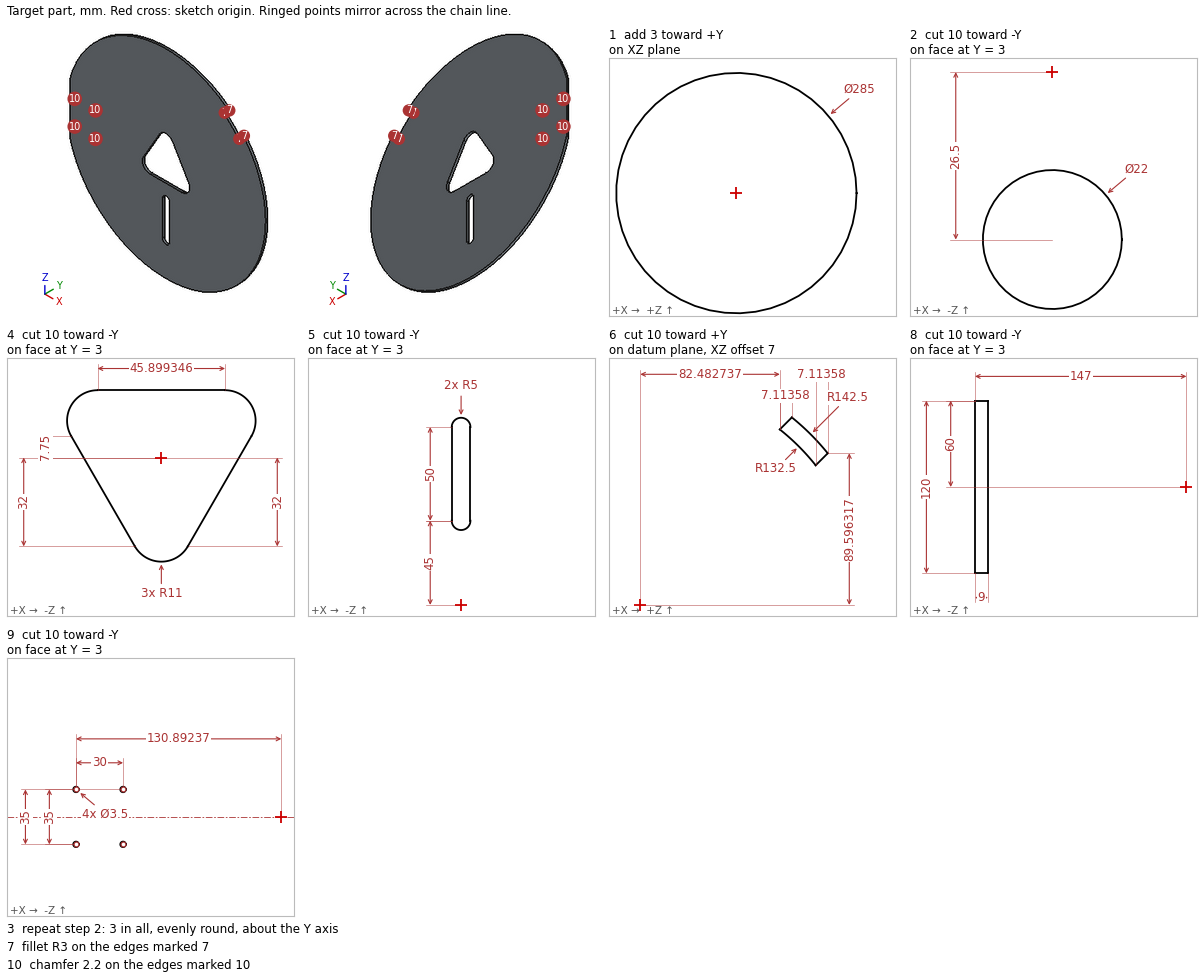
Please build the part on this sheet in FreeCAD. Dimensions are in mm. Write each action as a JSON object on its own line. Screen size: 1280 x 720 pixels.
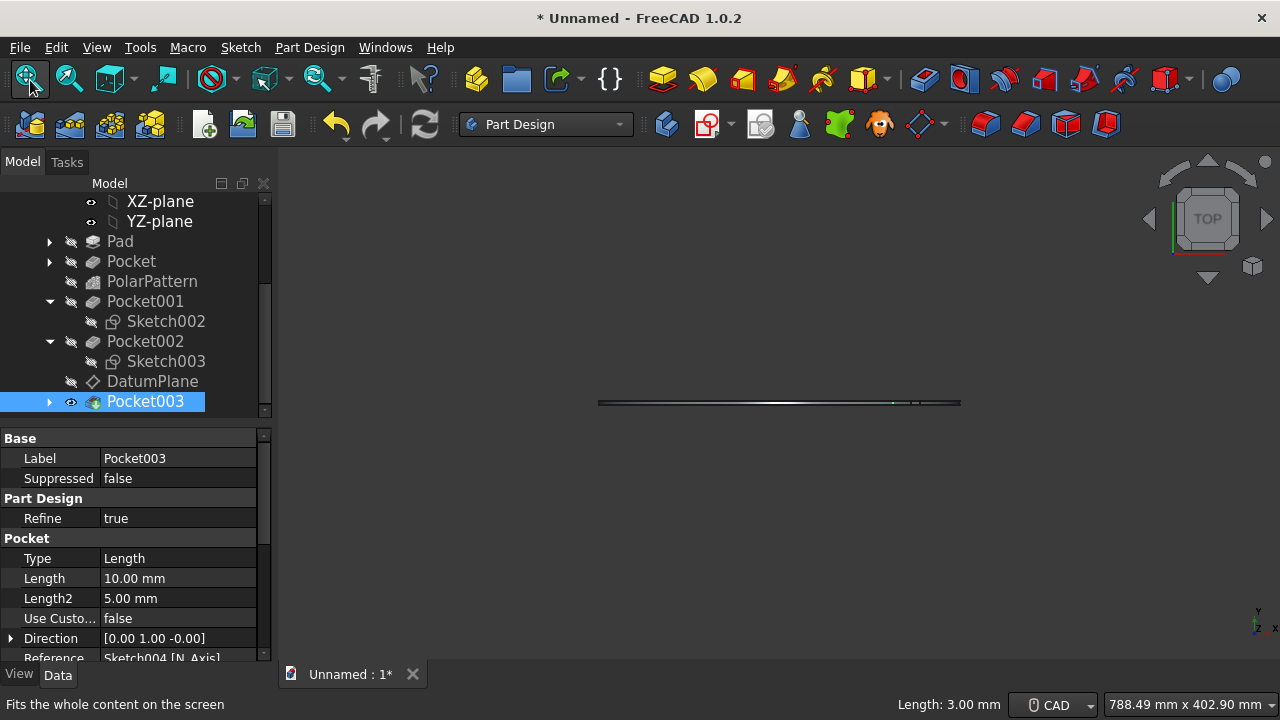
{"action": "key", "text": "1"}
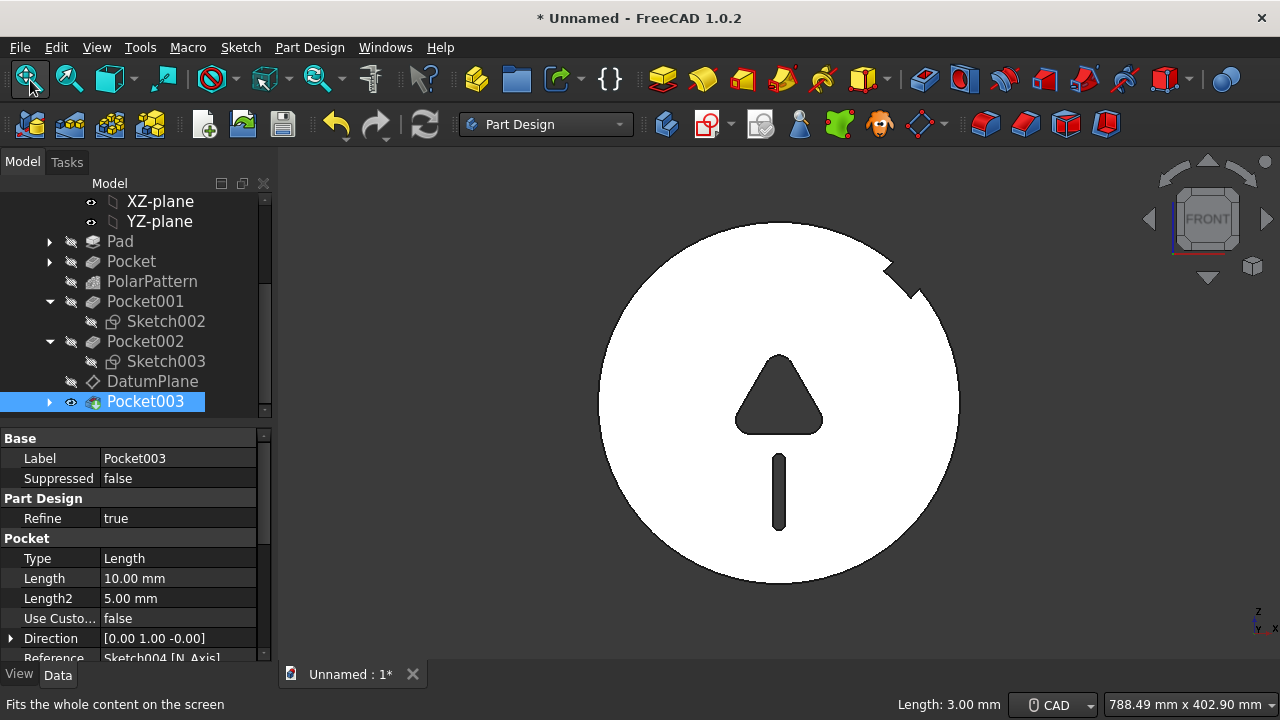
{"action": "scroll", "coordinate": [884, 270], "scroll_direction": "up", "scroll_amount": 12}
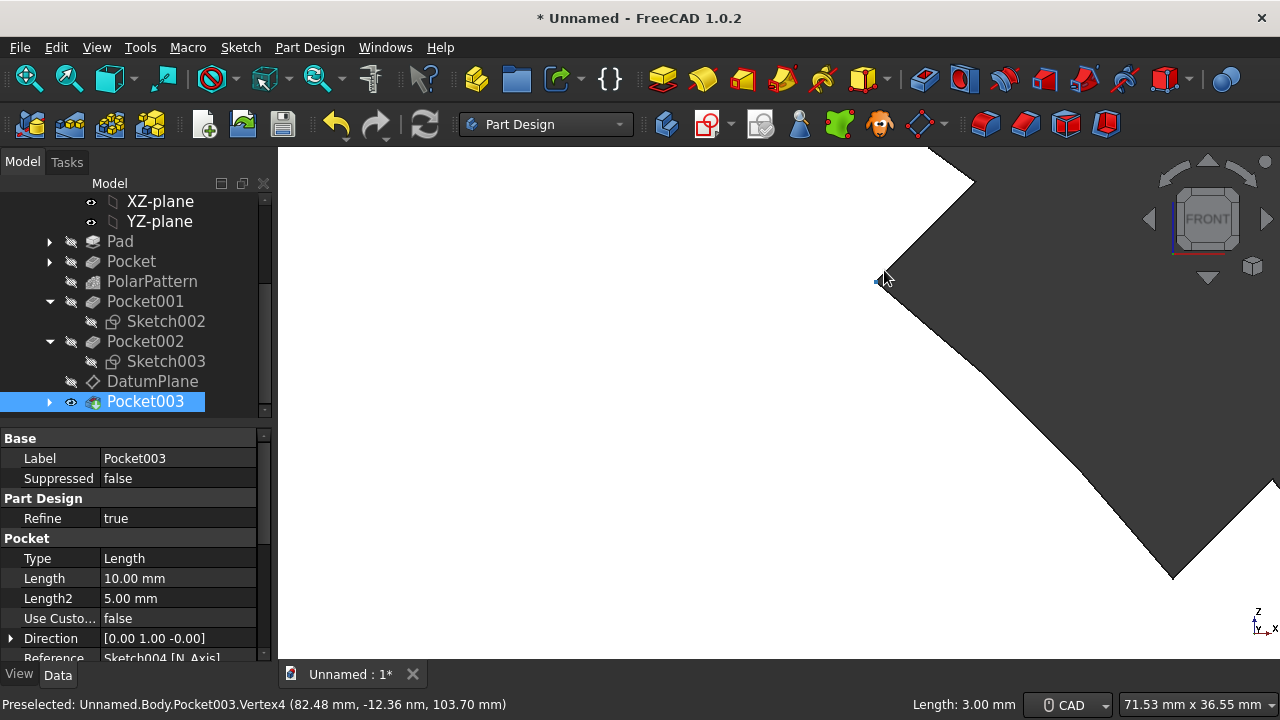
{"action": "left_click", "coordinate": [30, 80]}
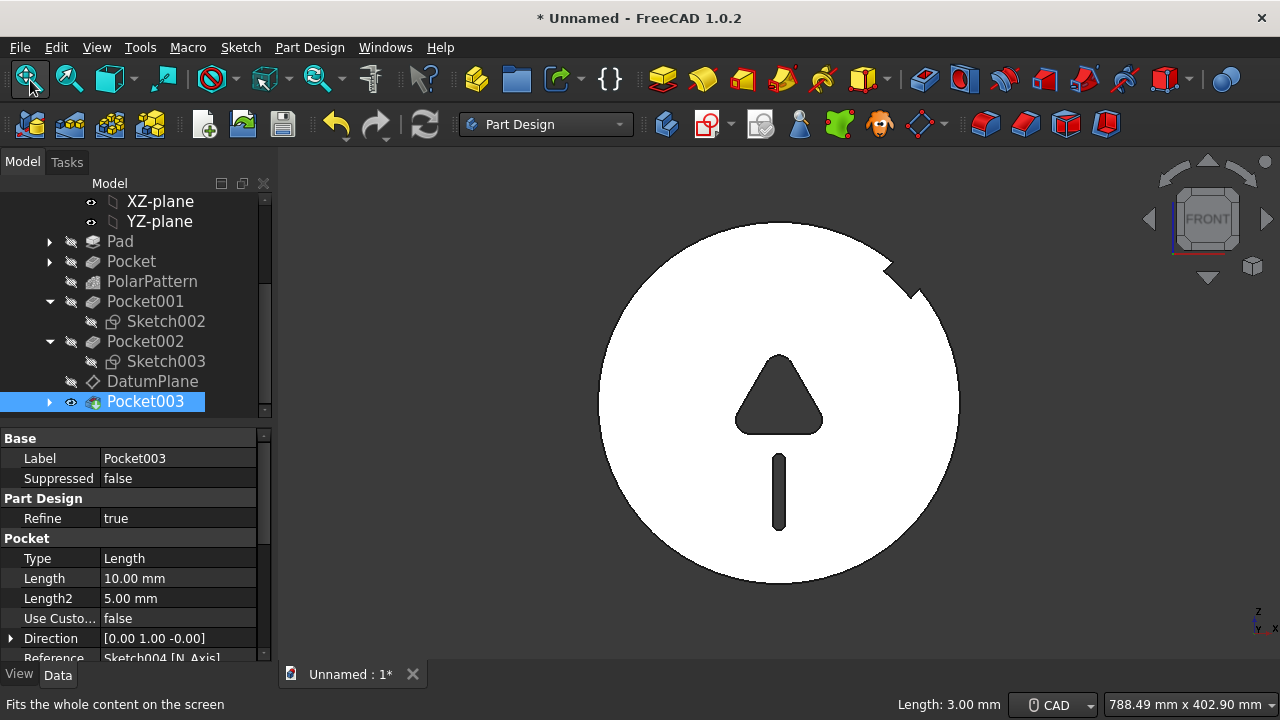
{"action": "key", "text": "3"}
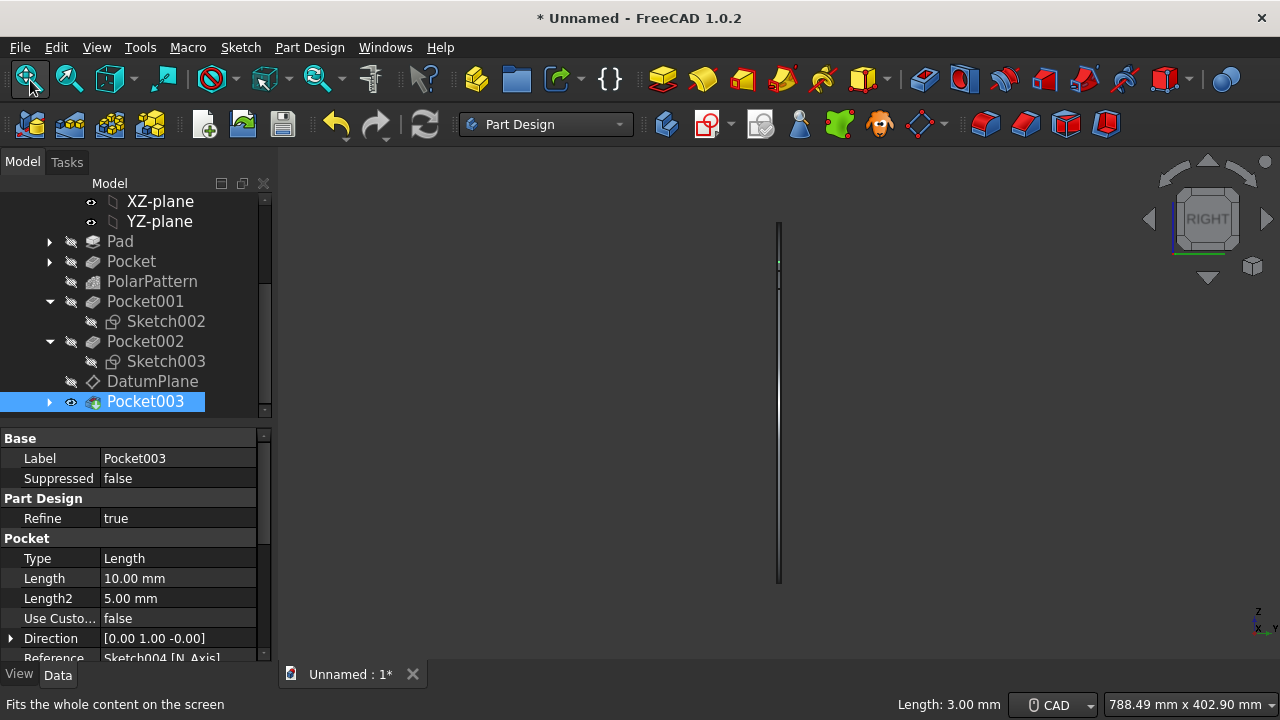
{"action": "scroll", "coordinate": [779, 270], "scroll_direction": "up", "scroll_amount": 12}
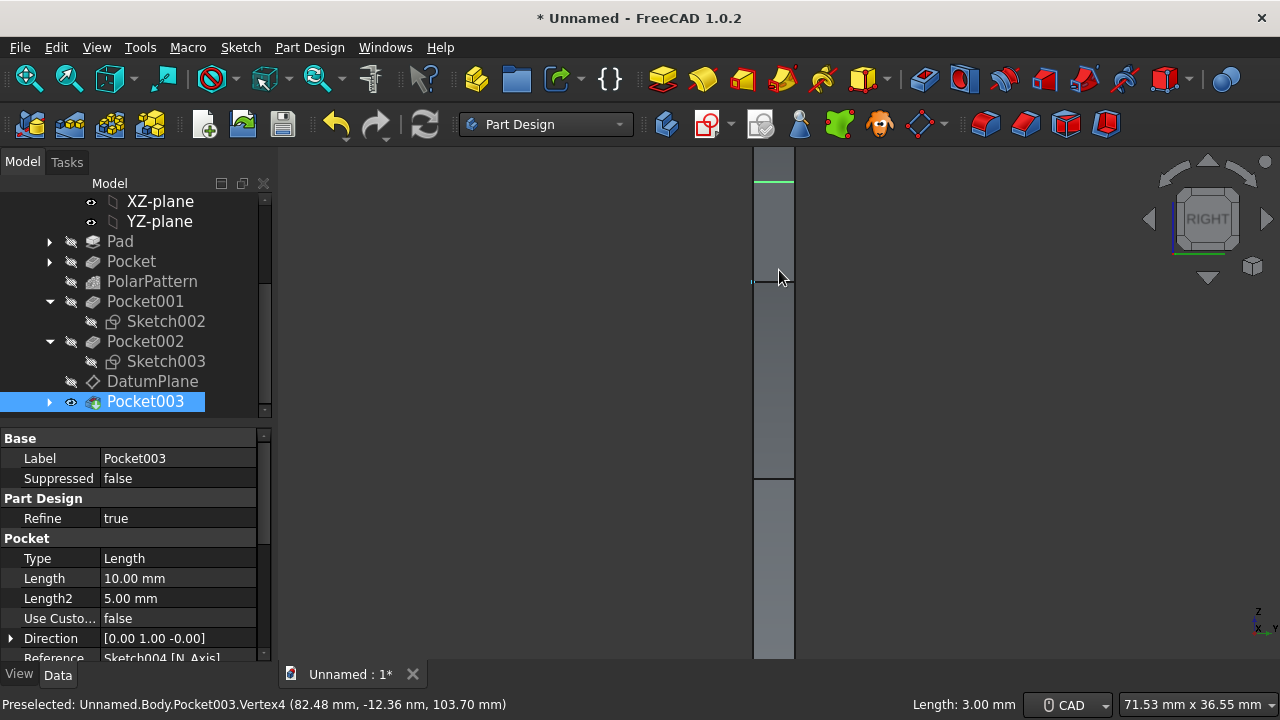
{"action": "left_click", "coordinate": [30, 80]}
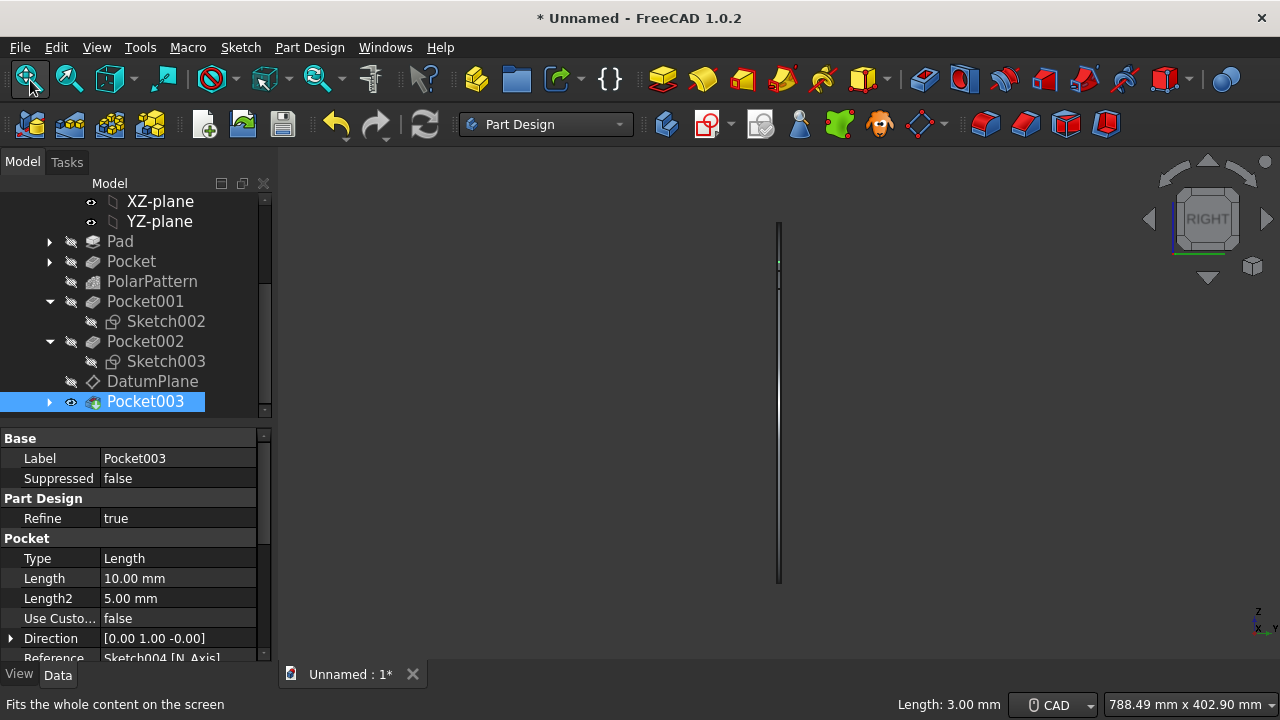
{"action": "key", "text": "5"}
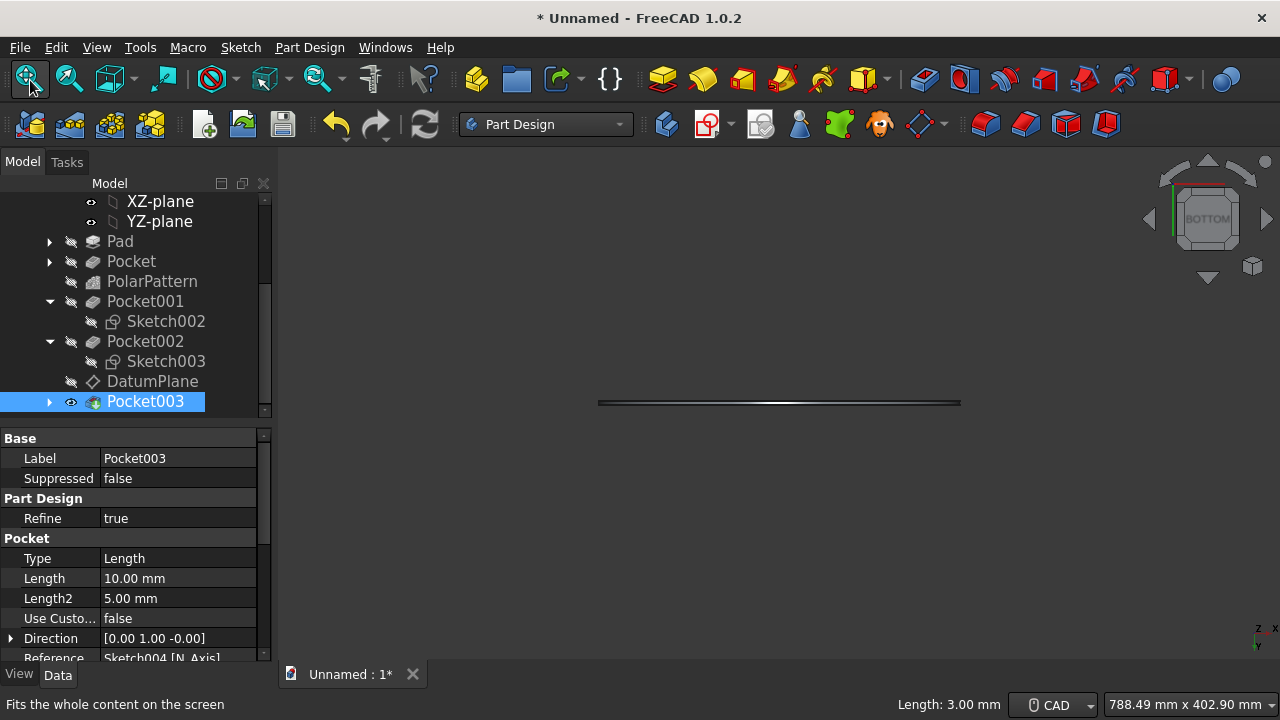
{"action": "key", "text": "v f"}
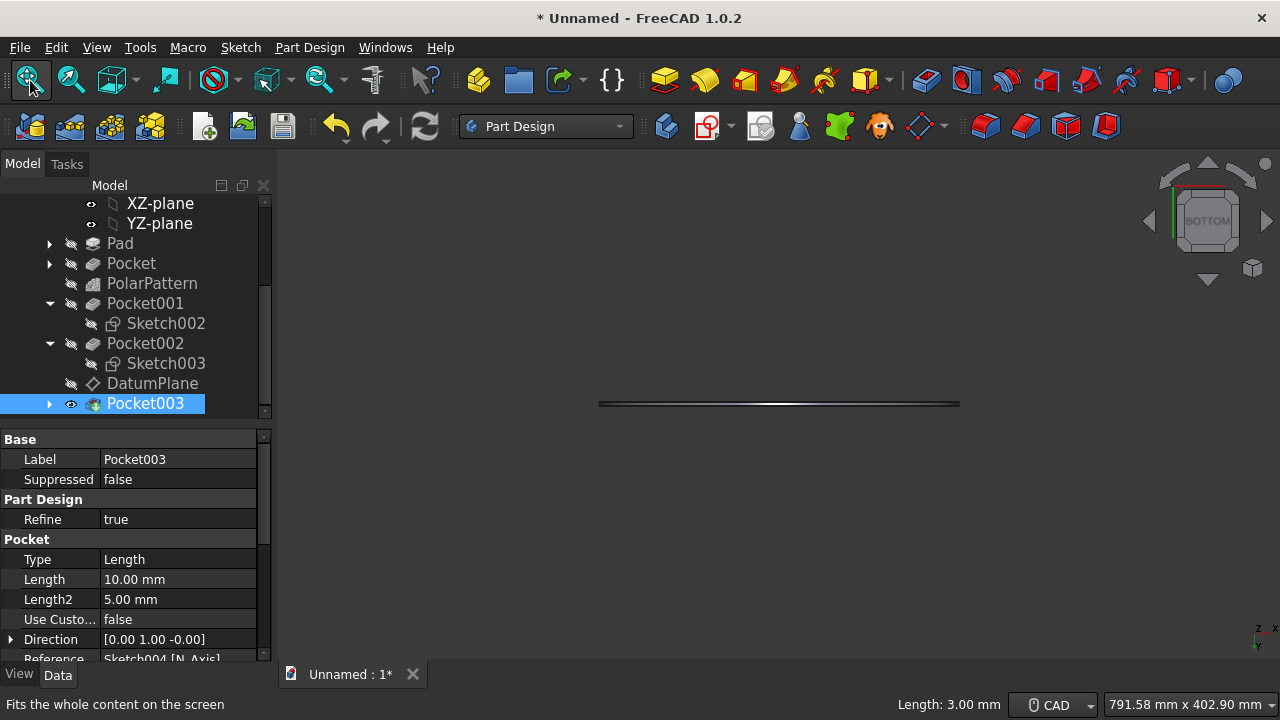
{"action": "scroll", "coordinate": [883, 403], "scroll_direction": "up", "scroll_amount": 12}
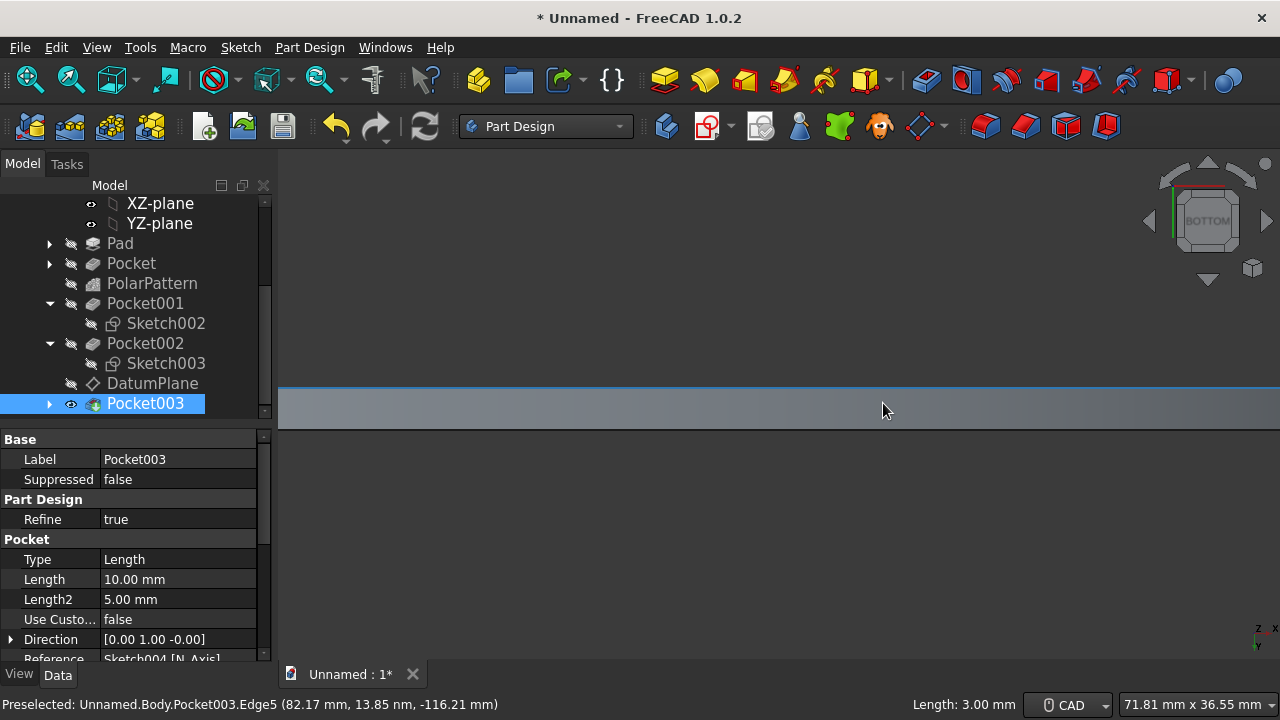
{"action": "left_click", "coordinate": [32, 80]}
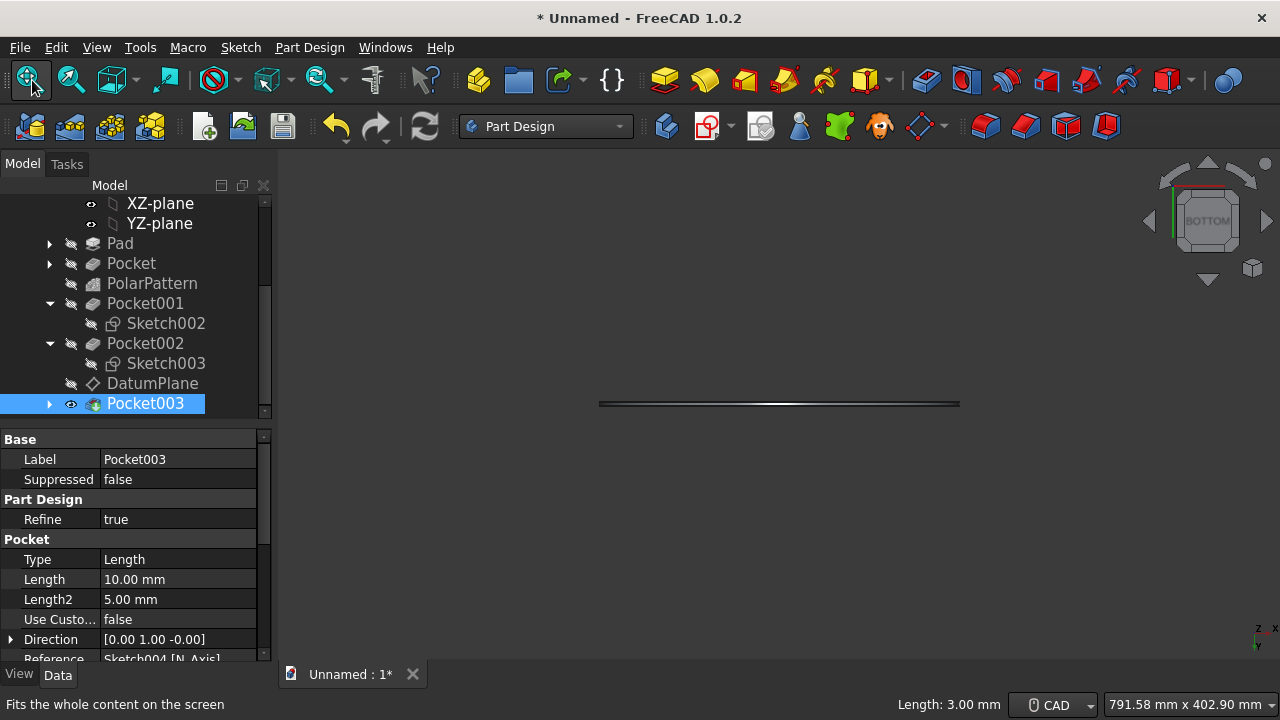
{"action": "key", "text": "4"}